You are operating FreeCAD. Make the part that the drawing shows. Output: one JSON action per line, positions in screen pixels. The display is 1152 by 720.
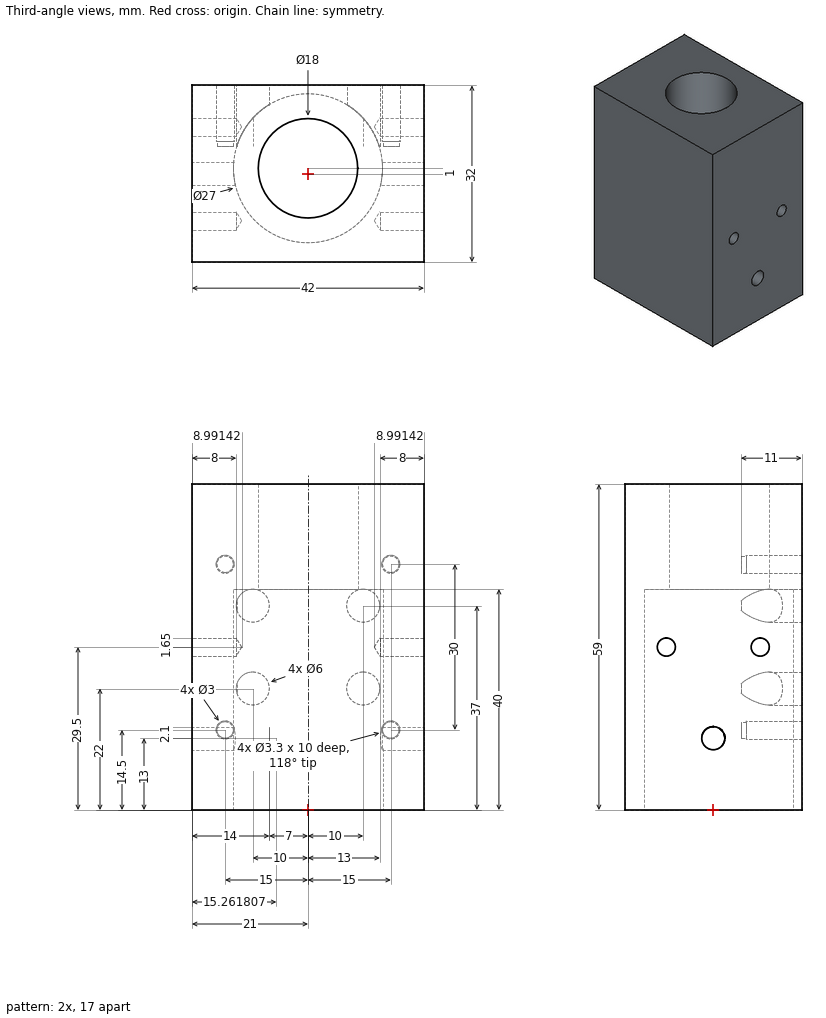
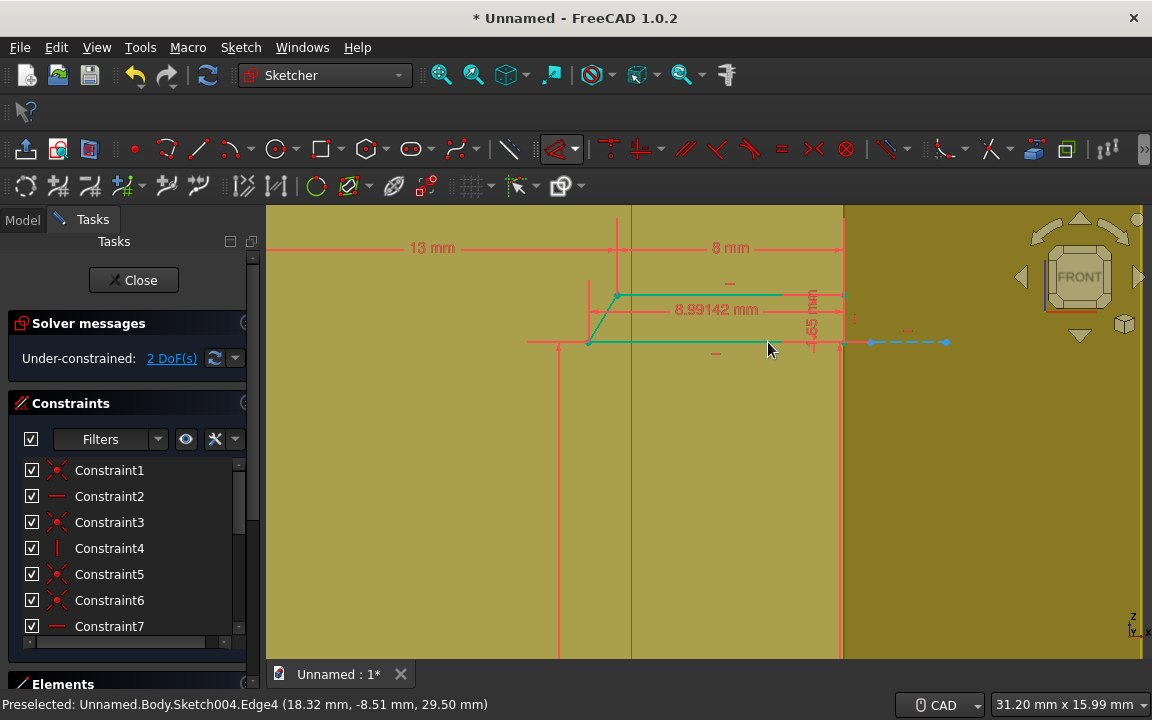
{"action": "left_click", "coordinate": [134, 280]}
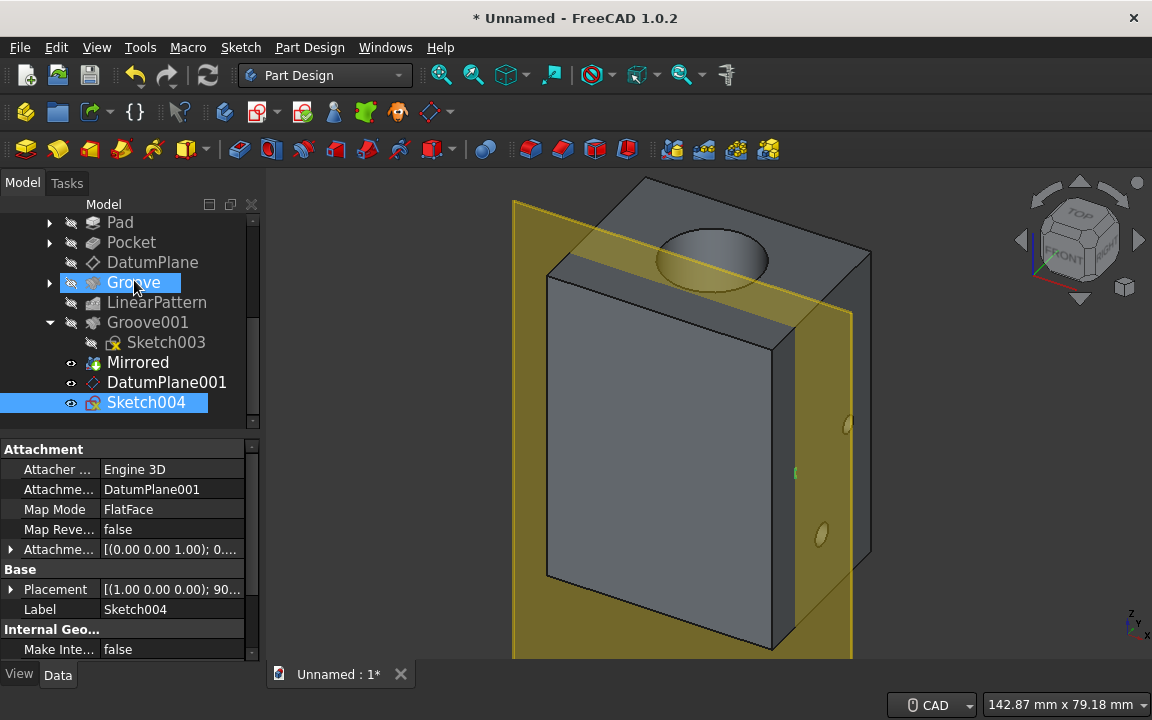
{"action": "left_click", "coordinate": [304, 150]}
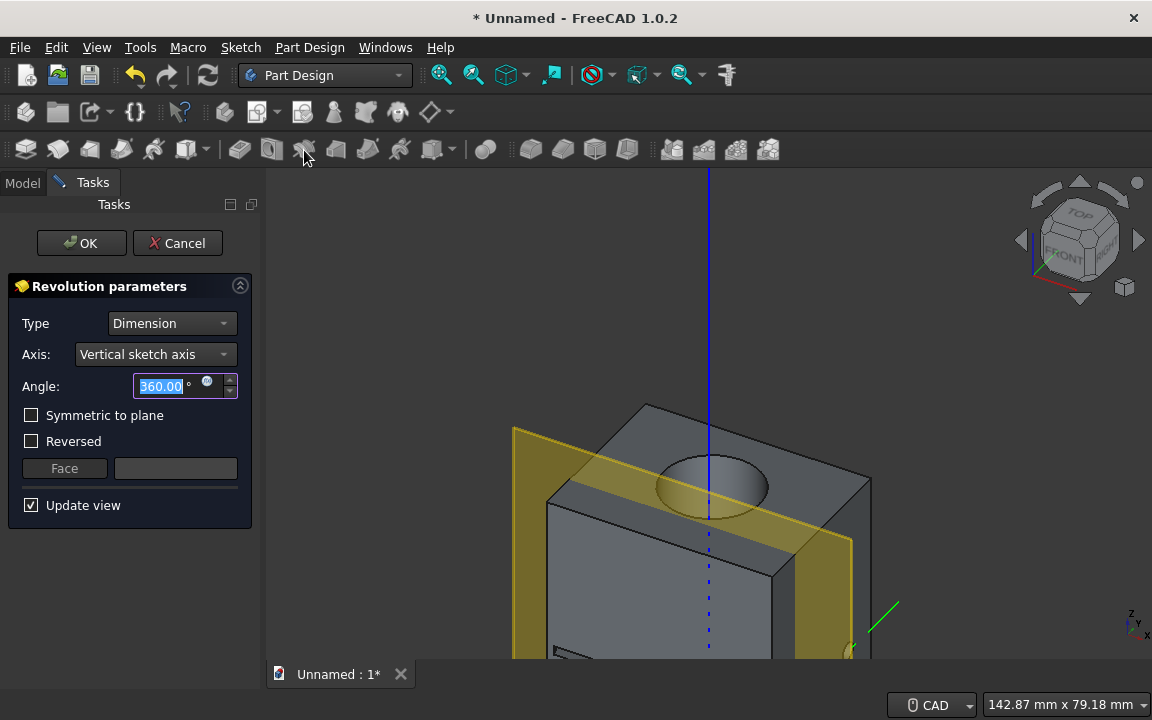
{"action": "left_click", "coordinate": [156, 354]}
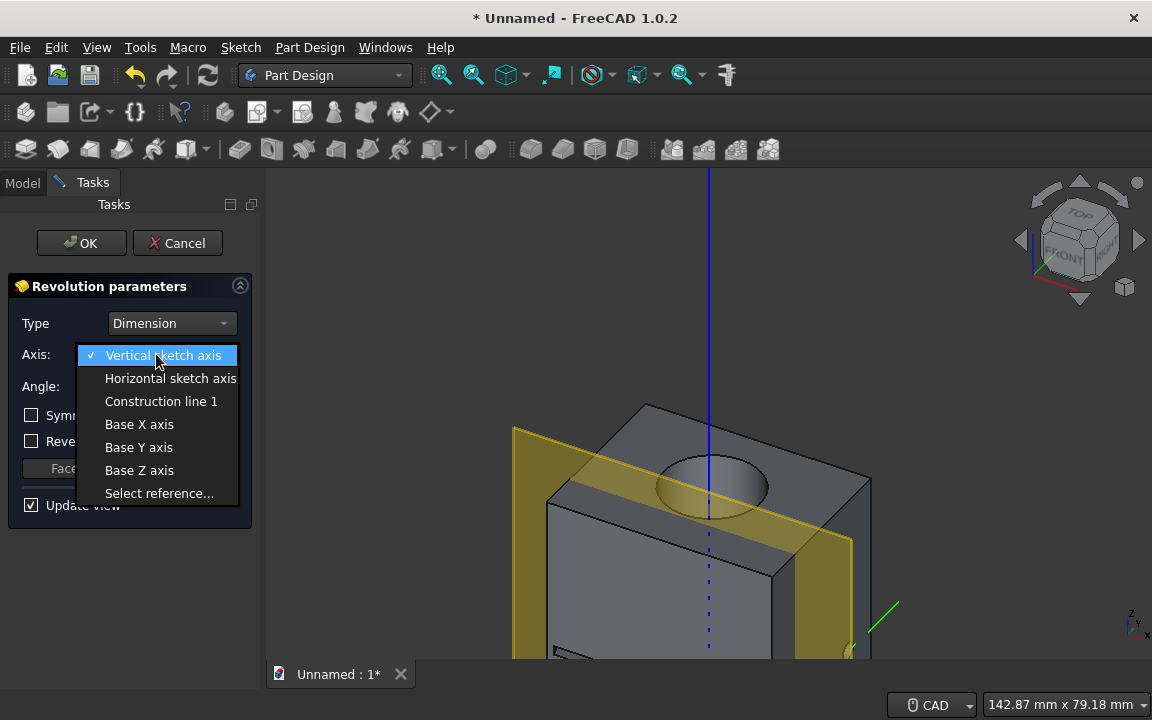
{"action": "left_click", "coordinate": [156, 402]}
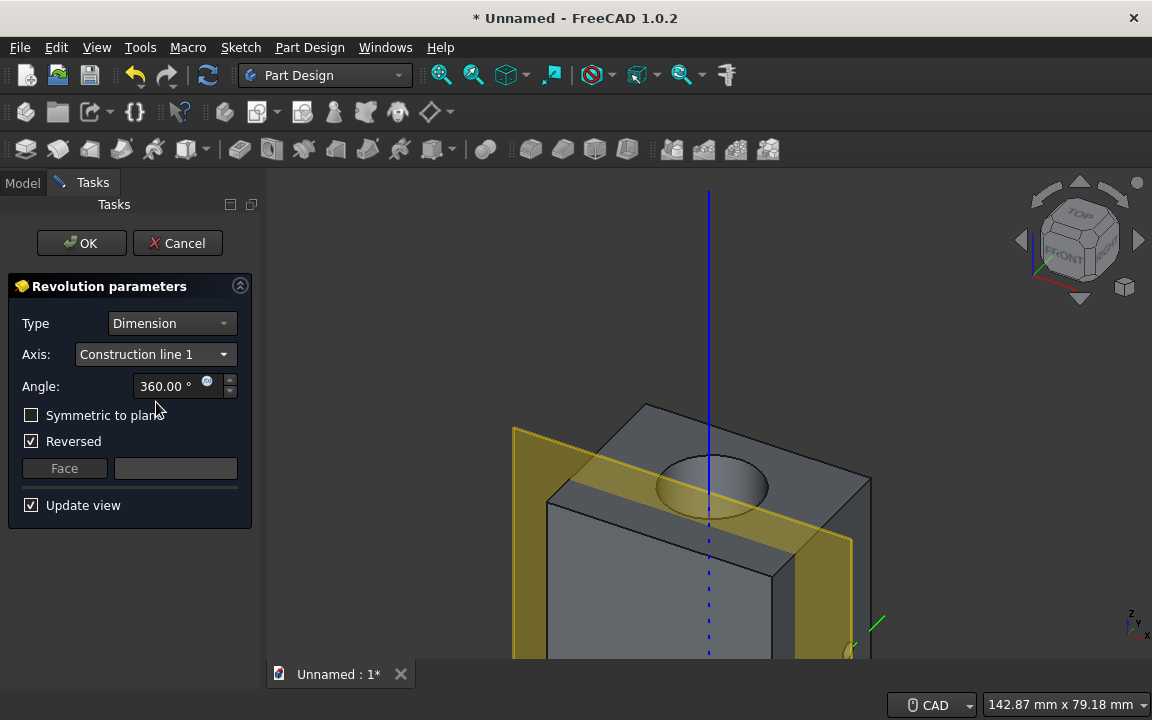
{"action": "left_click", "coordinate": [82, 243]}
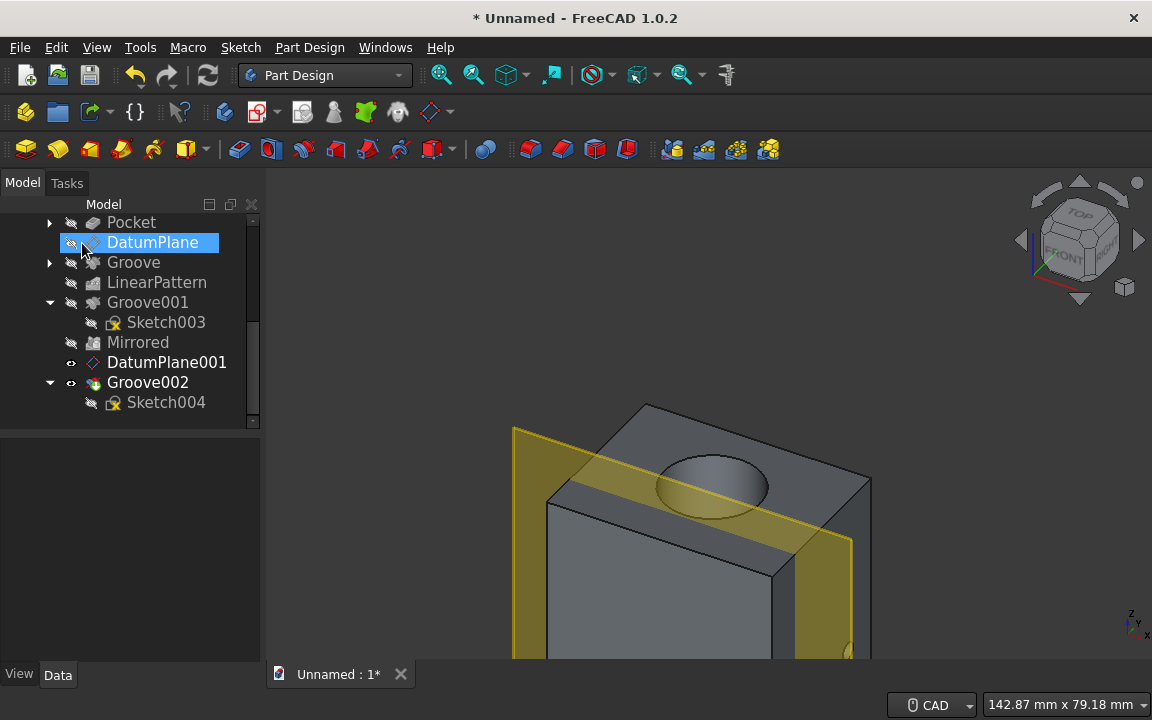
{"action": "left_click", "coordinate": [116, 363]}
{"action": "key", "text": "space"}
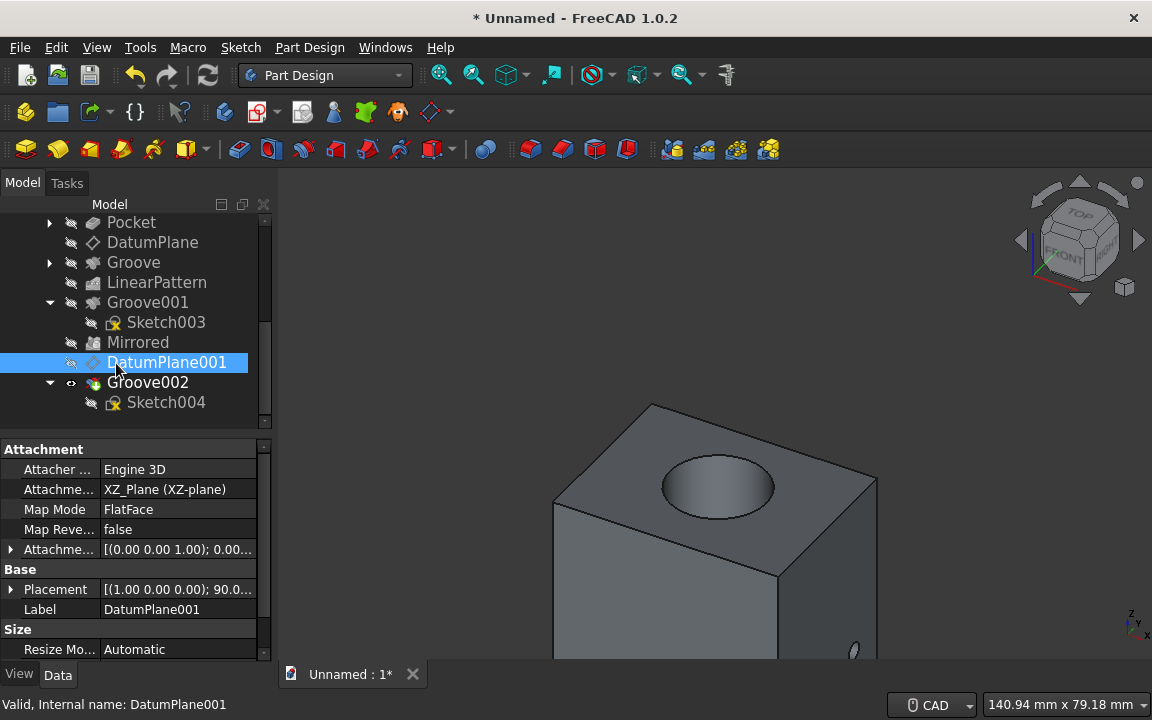
{"action": "key", "text": "v f"}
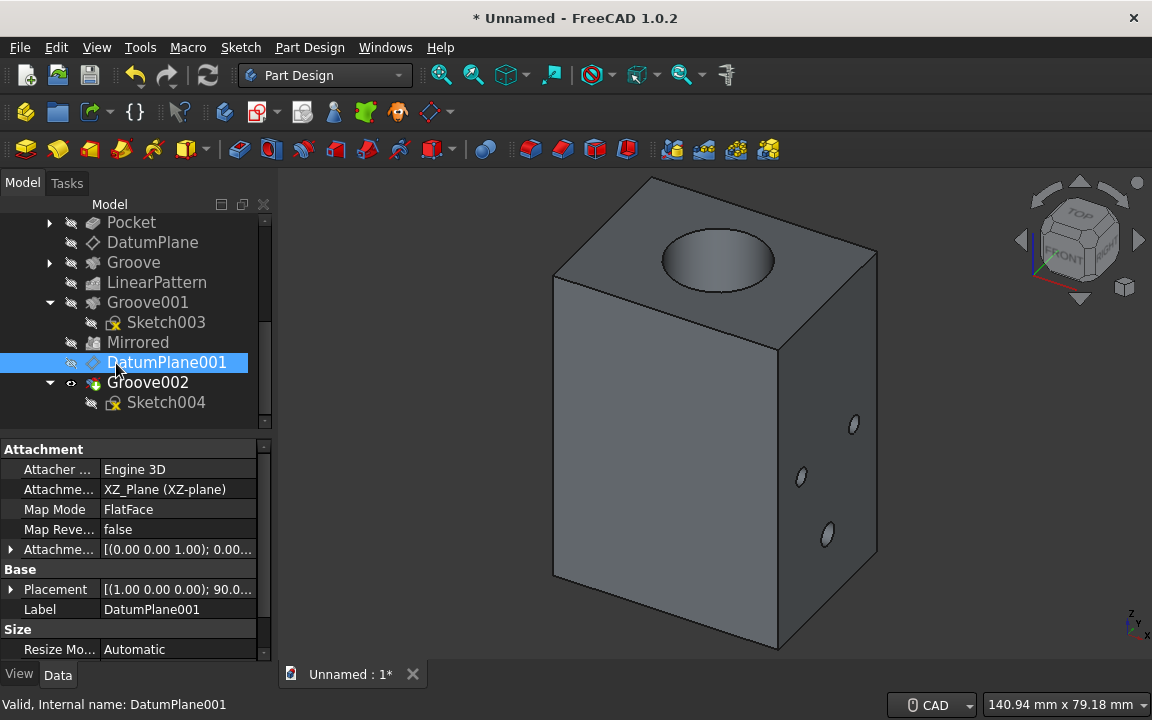
{"action": "key", "text": "4"}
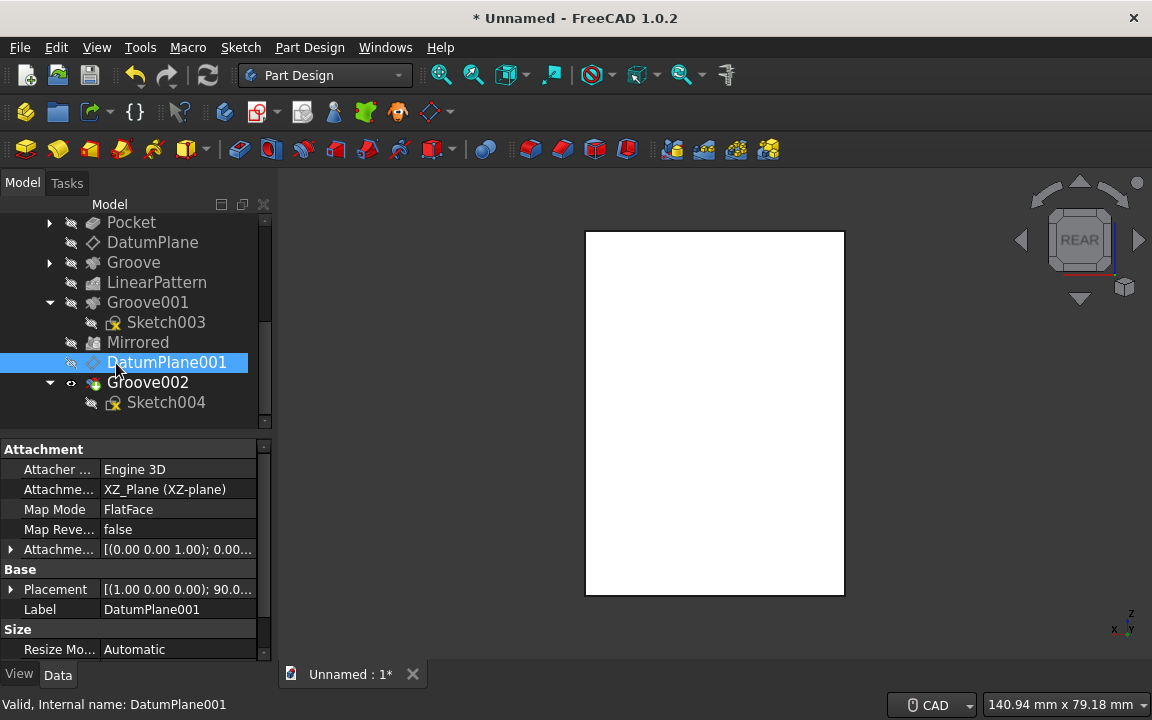
{"action": "left_click", "coordinate": [715, 360]}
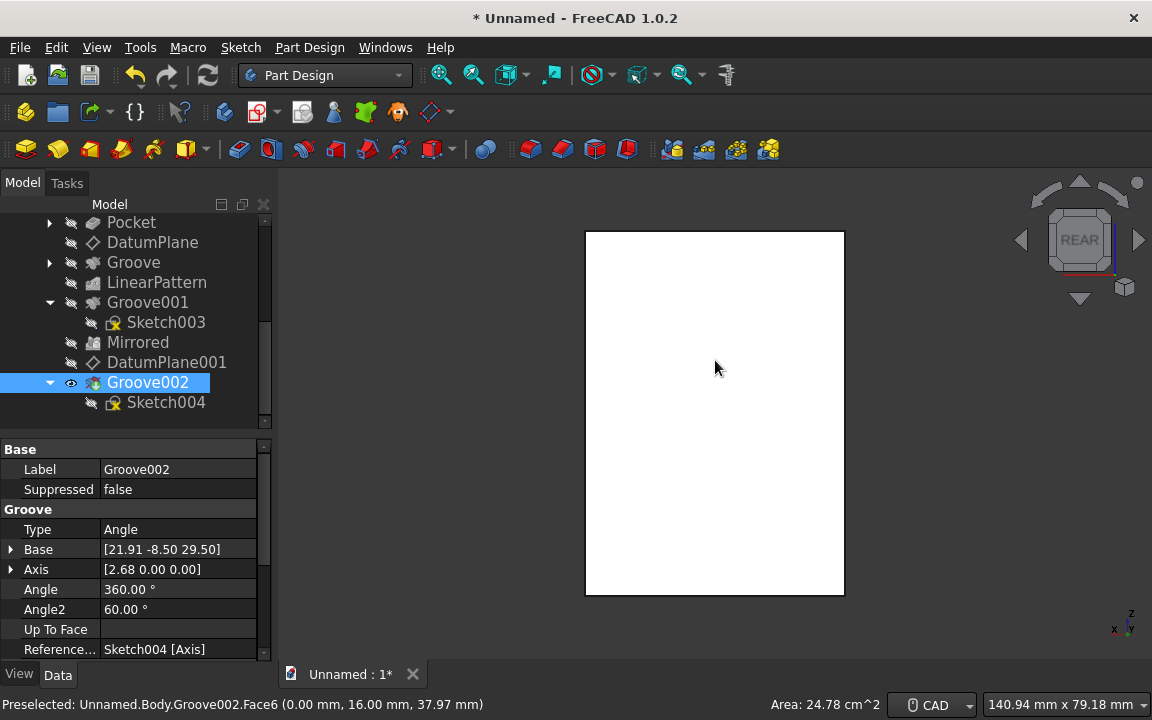
{"action": "left_click", "coordinate": [258, 112]}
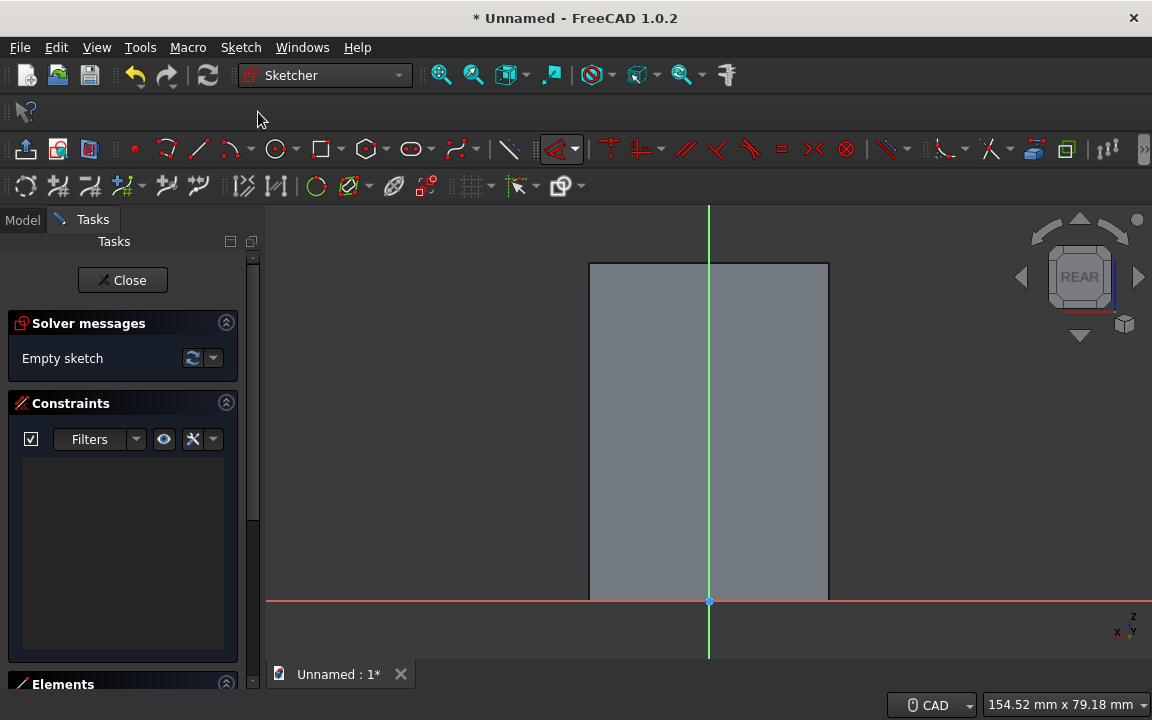
{"action": "key", "text": "g c"}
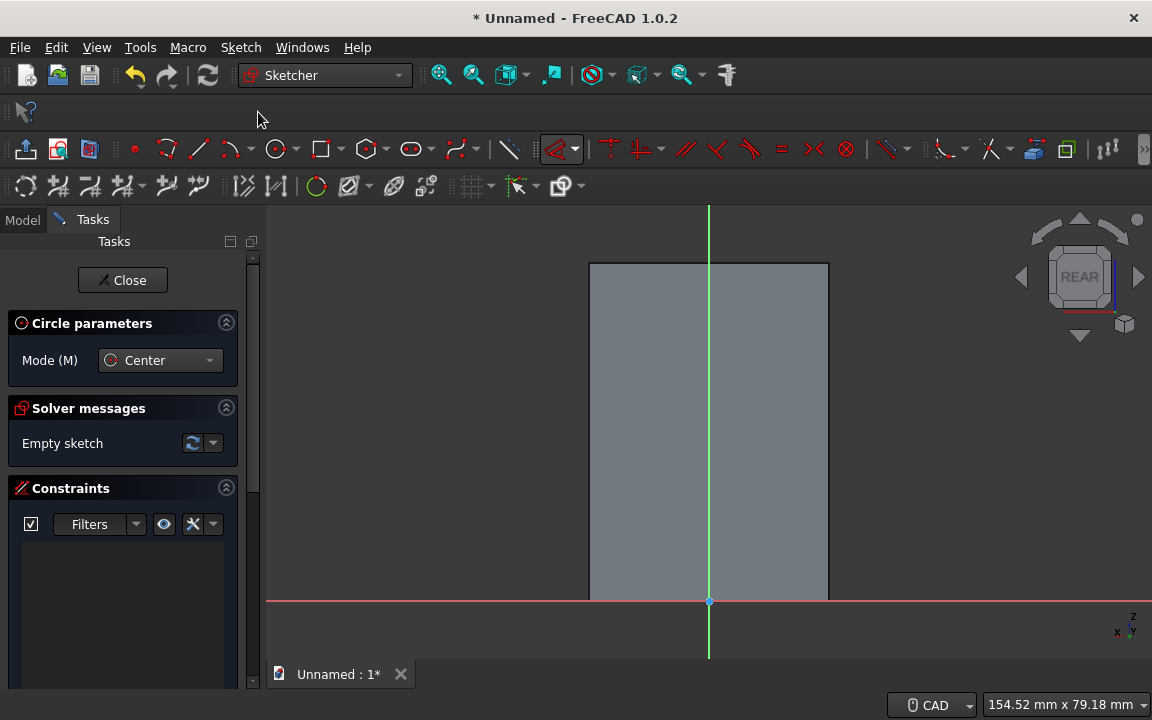
{"action": "scroll", "coordinate": [795, 518], "scroll_direction": "up", "scroll_amount": 5}